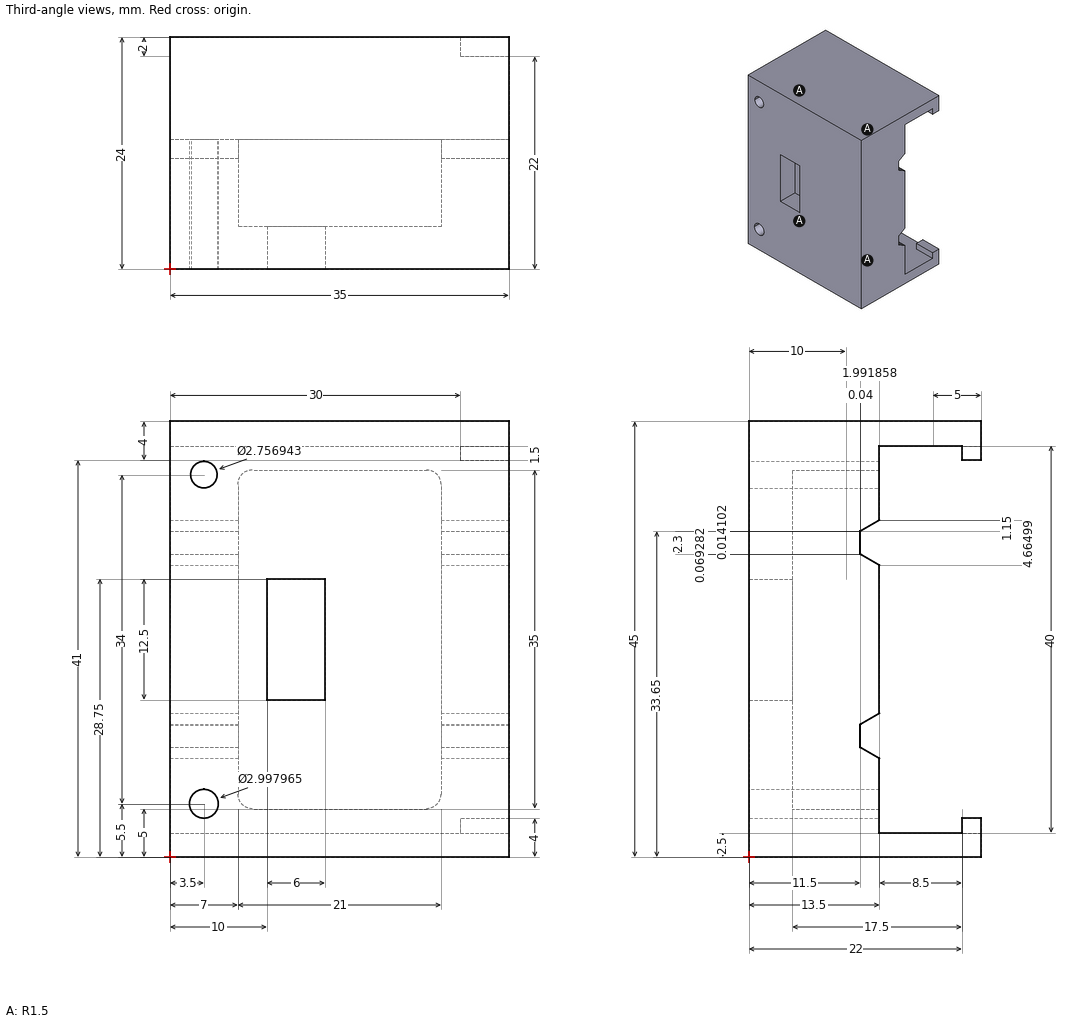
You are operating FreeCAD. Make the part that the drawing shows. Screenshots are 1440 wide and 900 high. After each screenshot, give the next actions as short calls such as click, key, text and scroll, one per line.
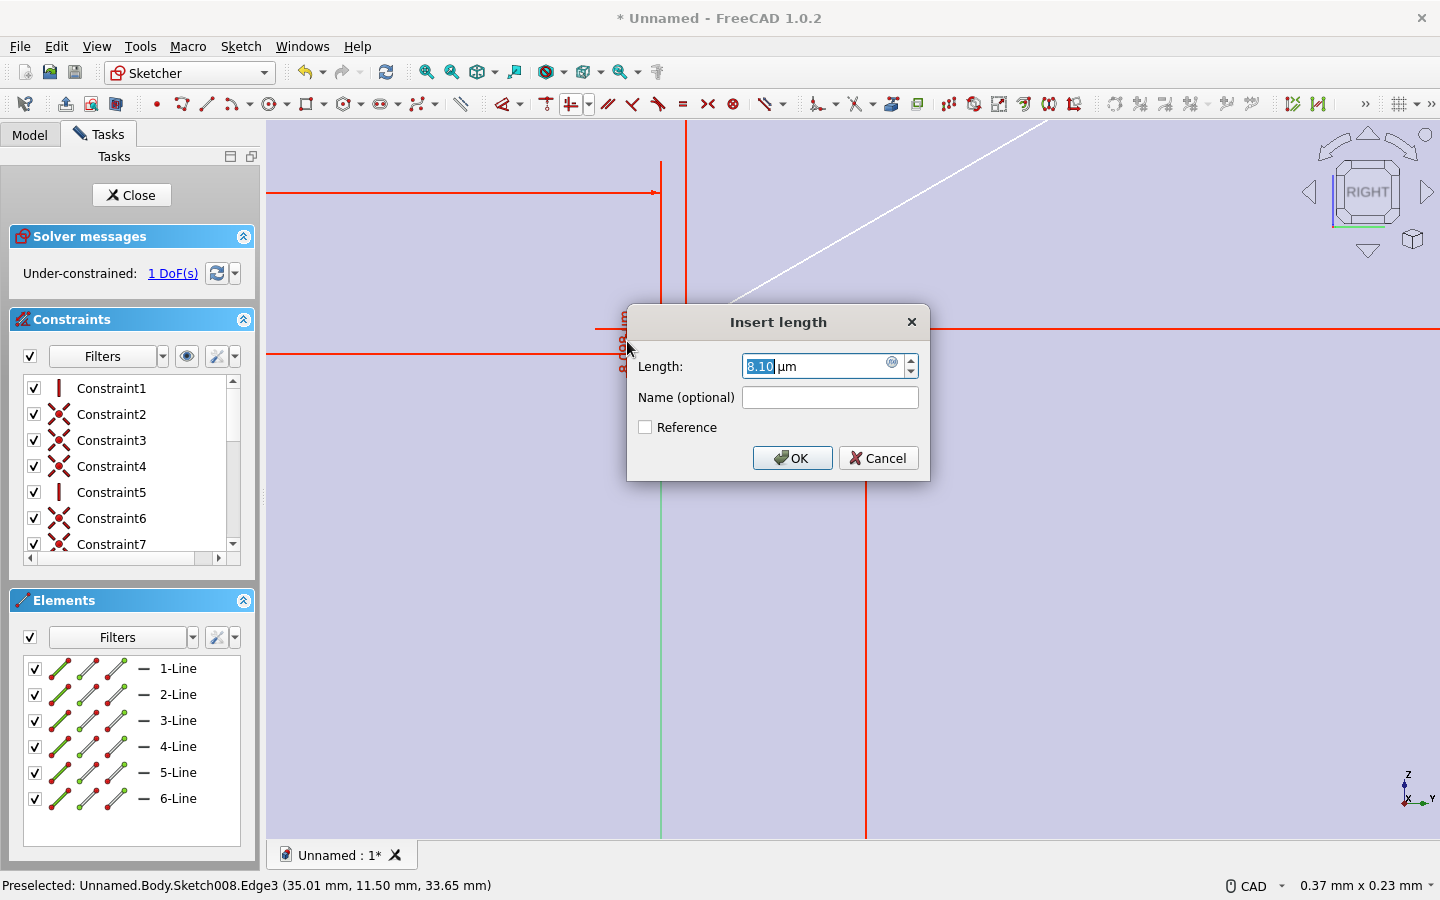
key(ctrl+a)
text(0.014102 mm)
key(Return)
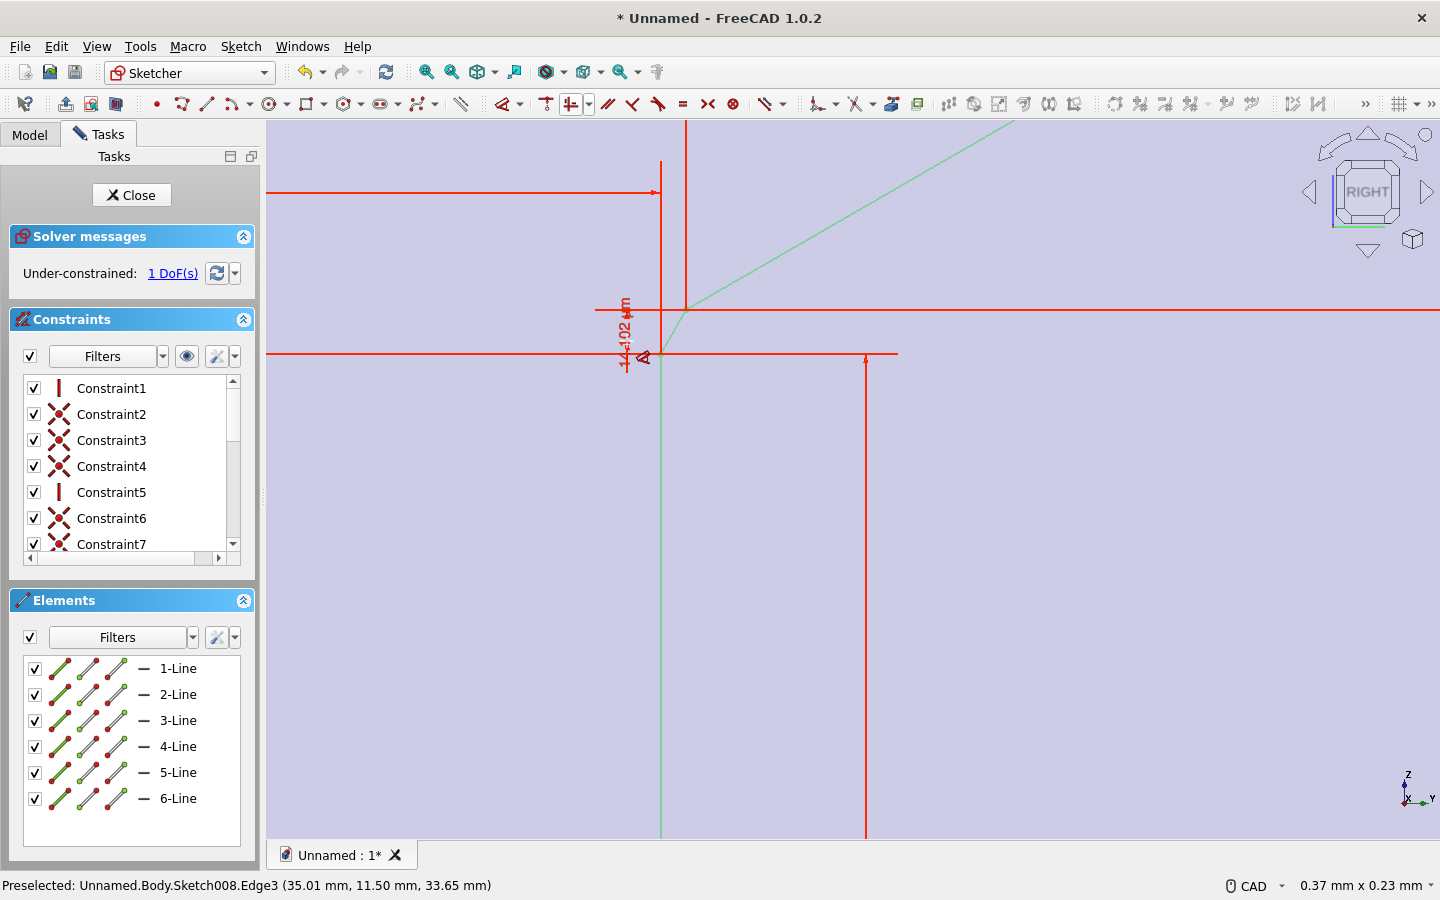
scroll(656, 329, down, 16)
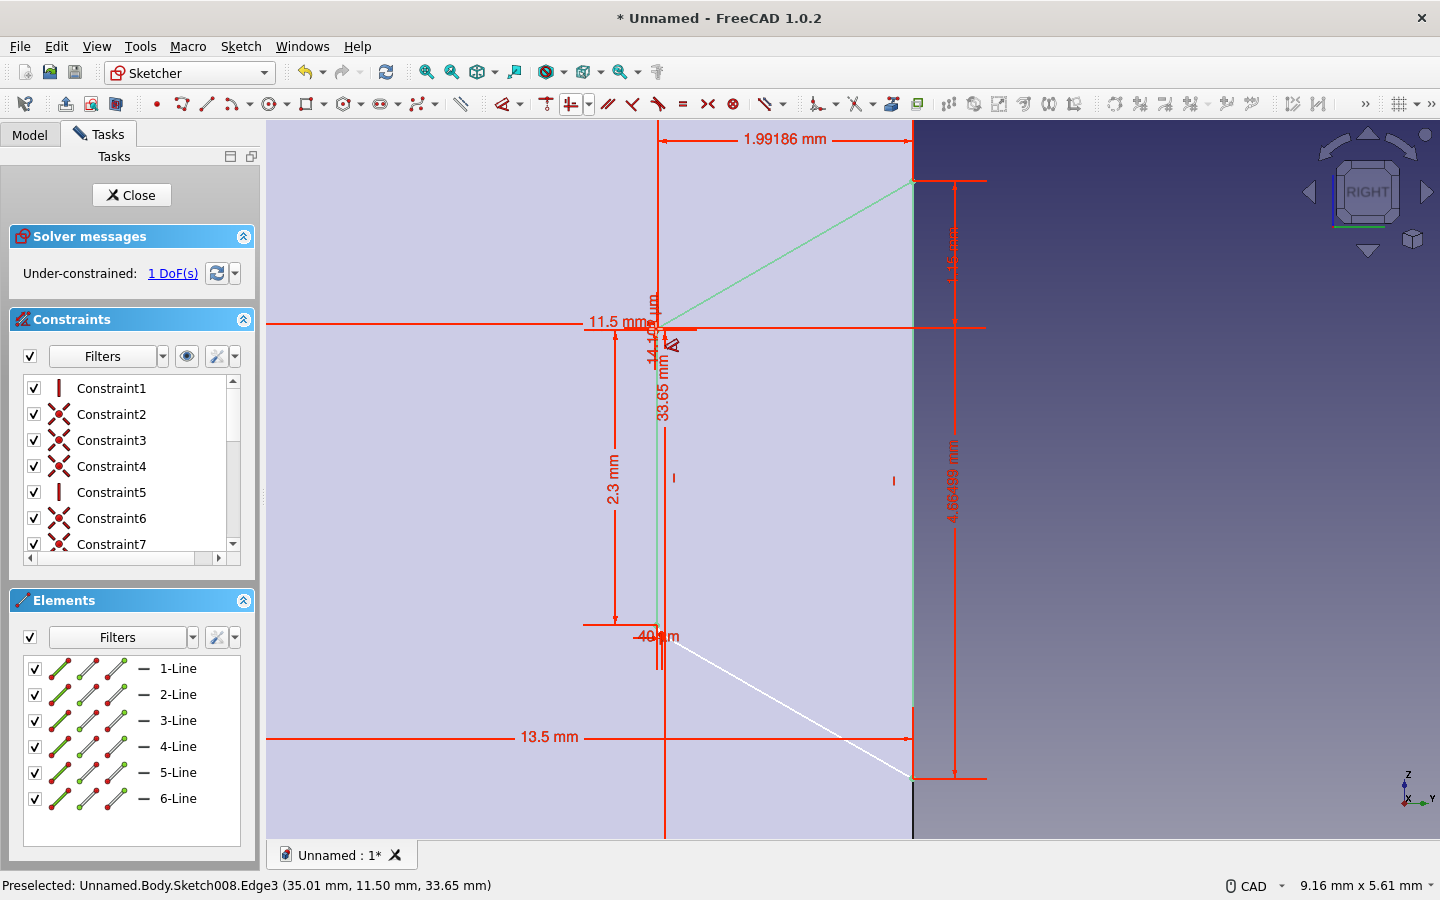
scroll(658, 628, up, 8)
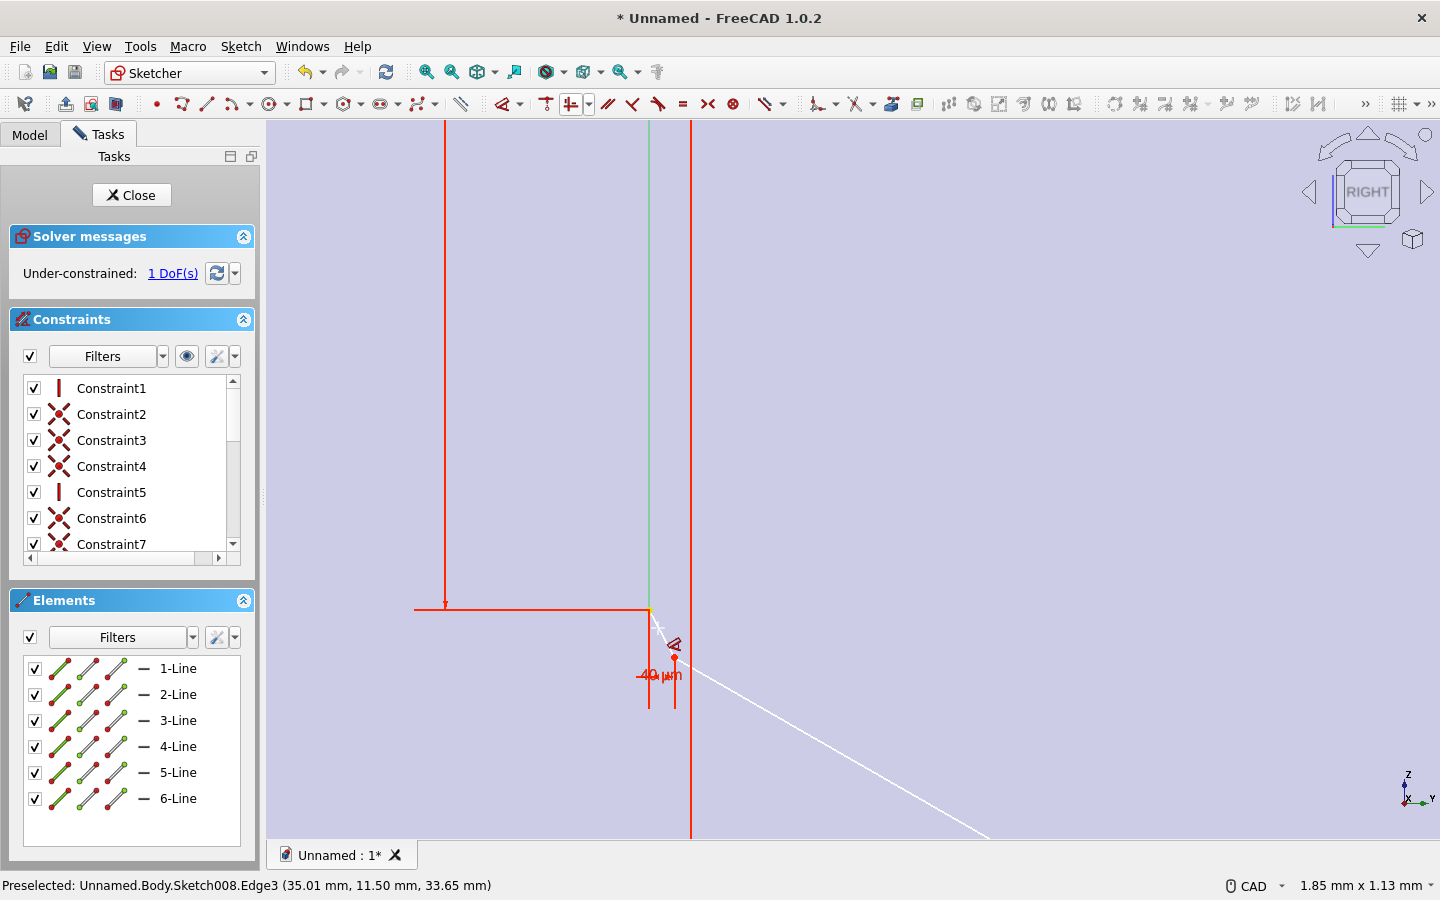
click(657, 625)
click(615, 634)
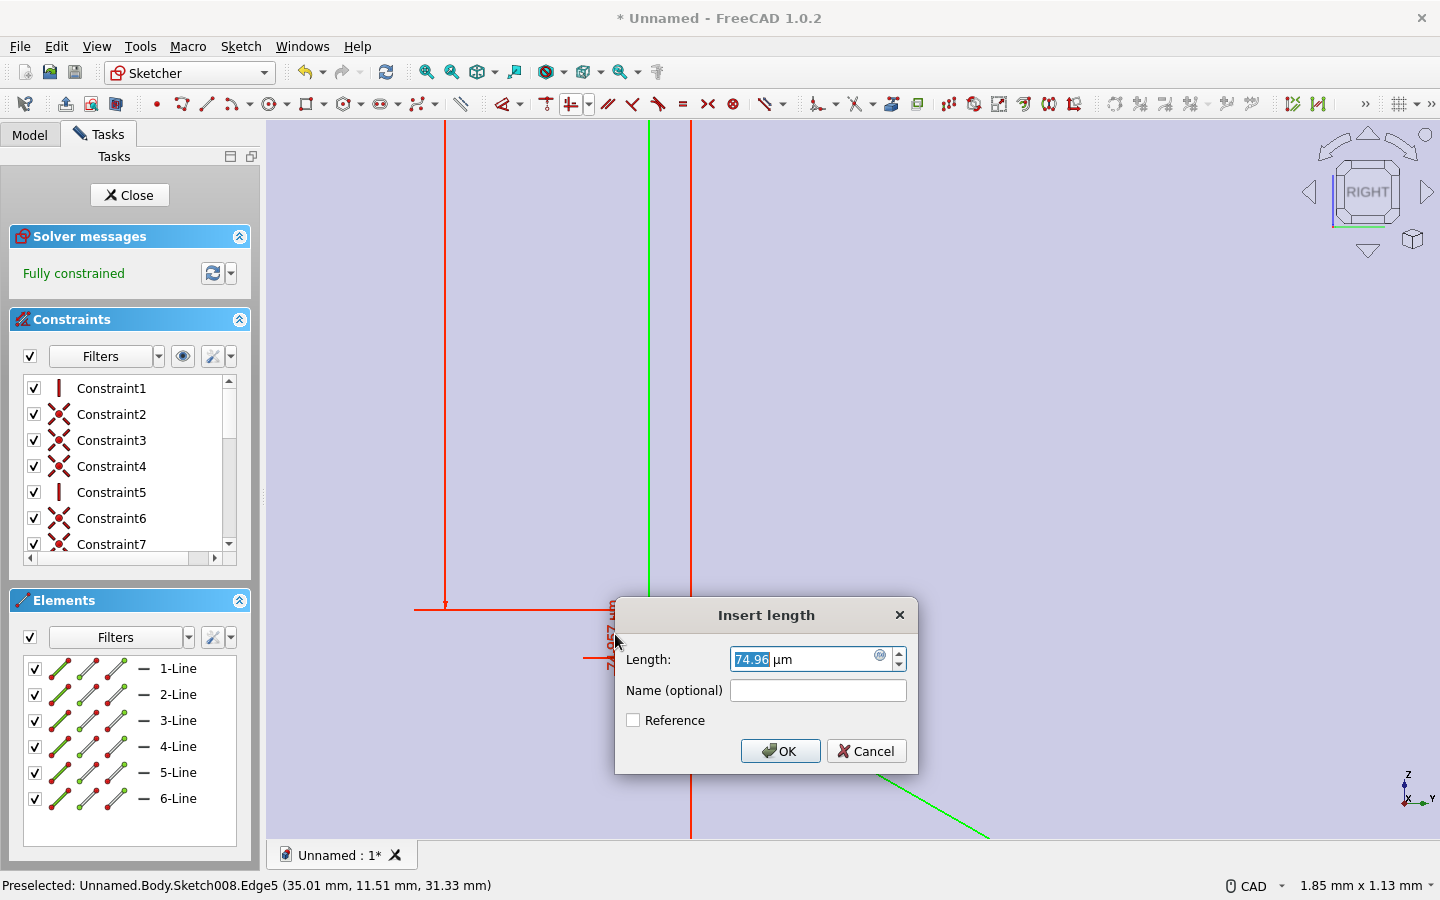
key(ctrl+a)
text(0.069282 mm)
key(Return)
key(Escape)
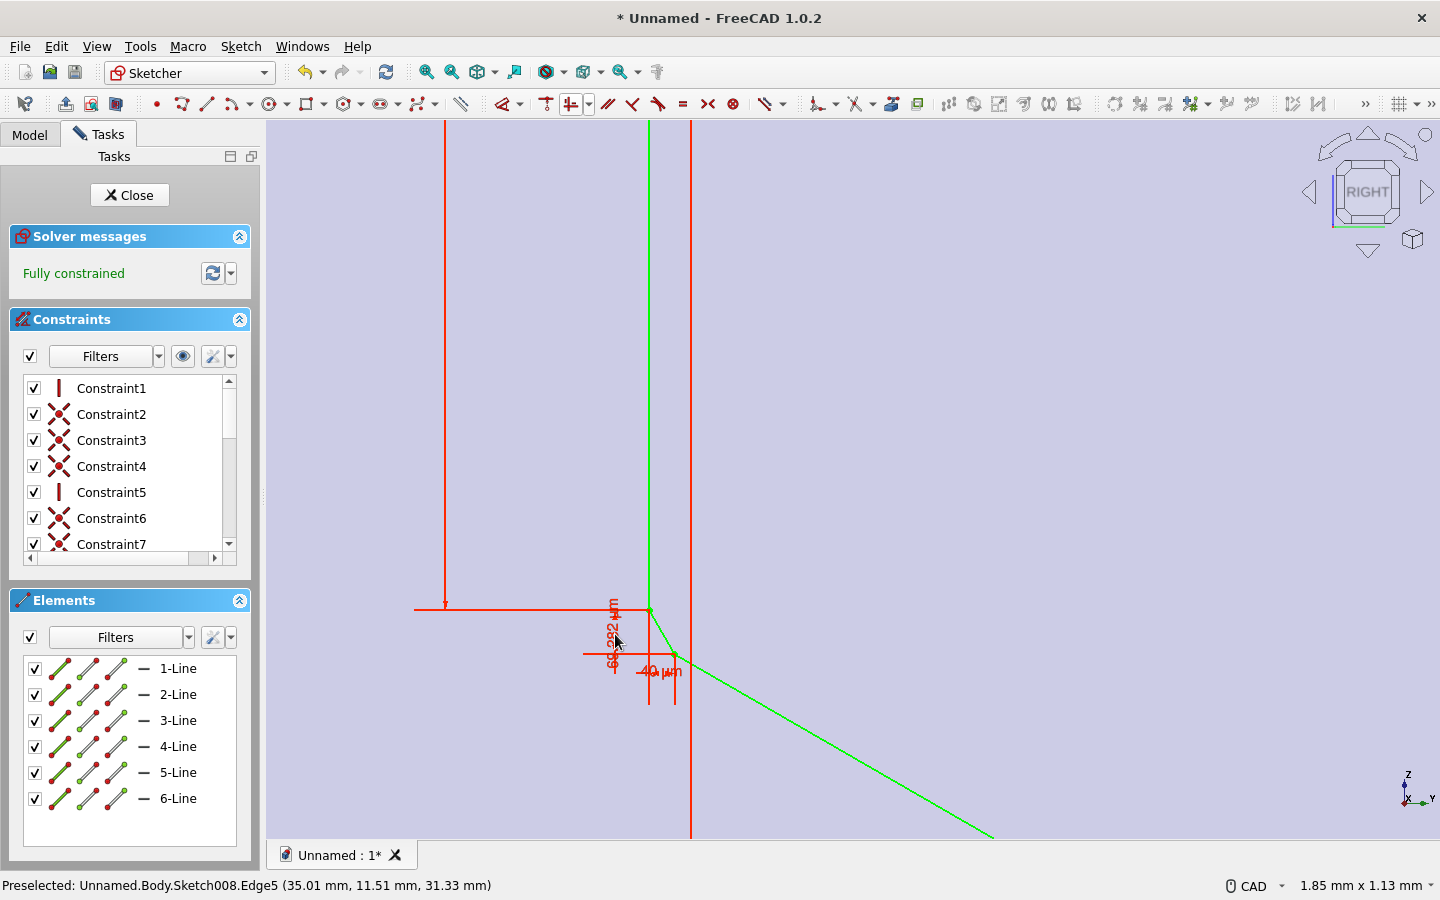
click(130, 195)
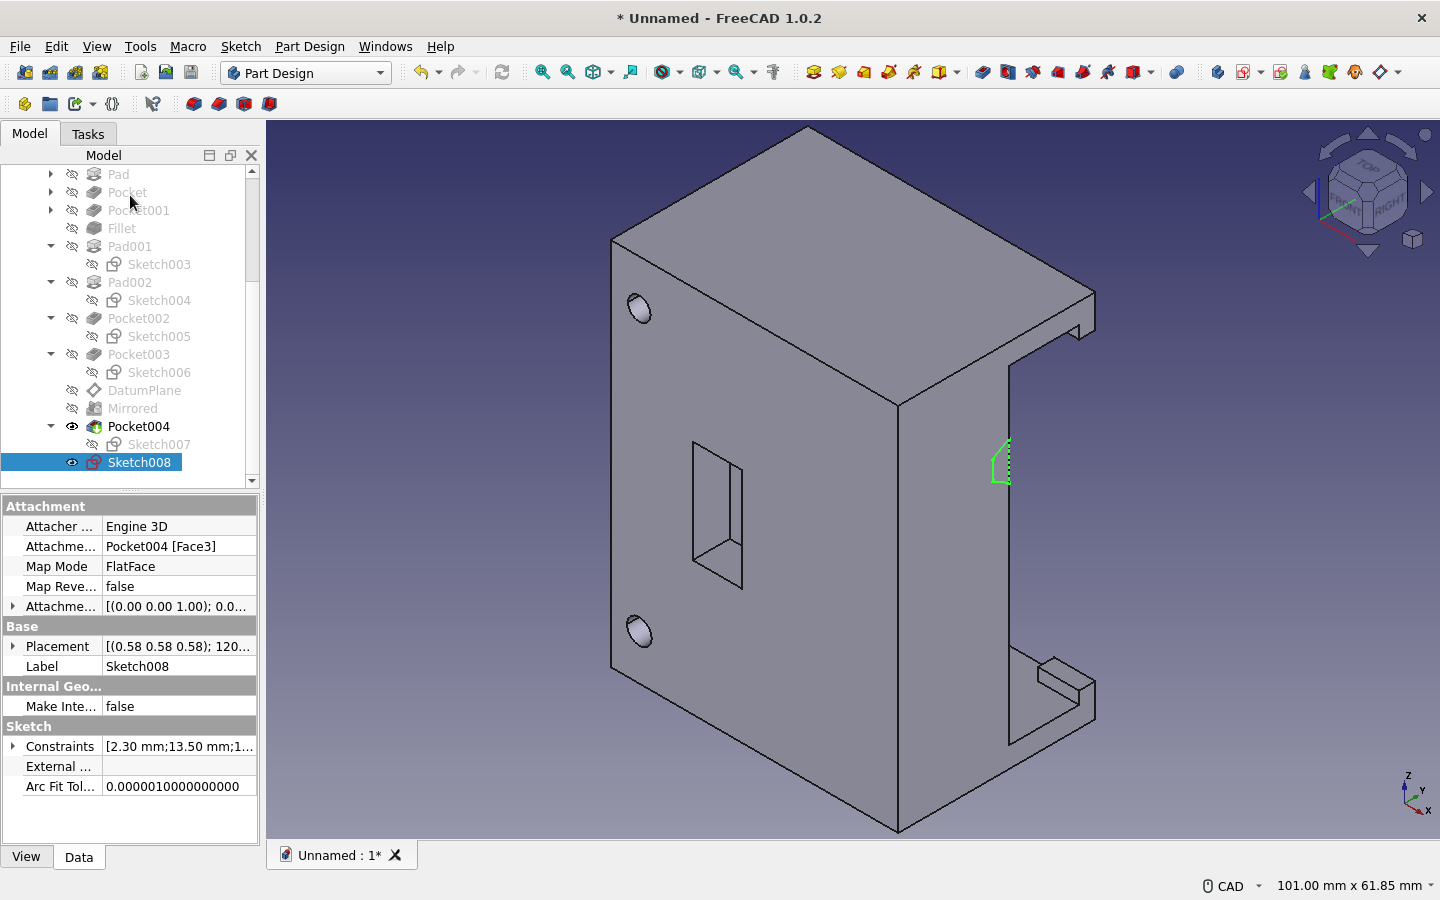
click(983, 72)